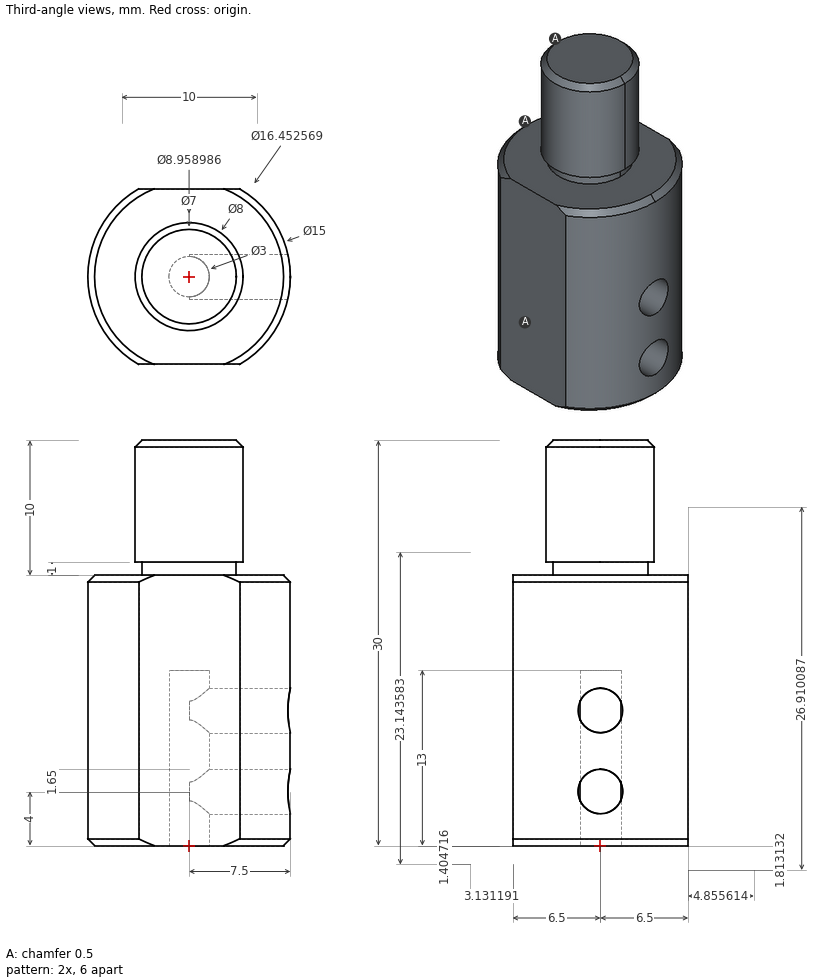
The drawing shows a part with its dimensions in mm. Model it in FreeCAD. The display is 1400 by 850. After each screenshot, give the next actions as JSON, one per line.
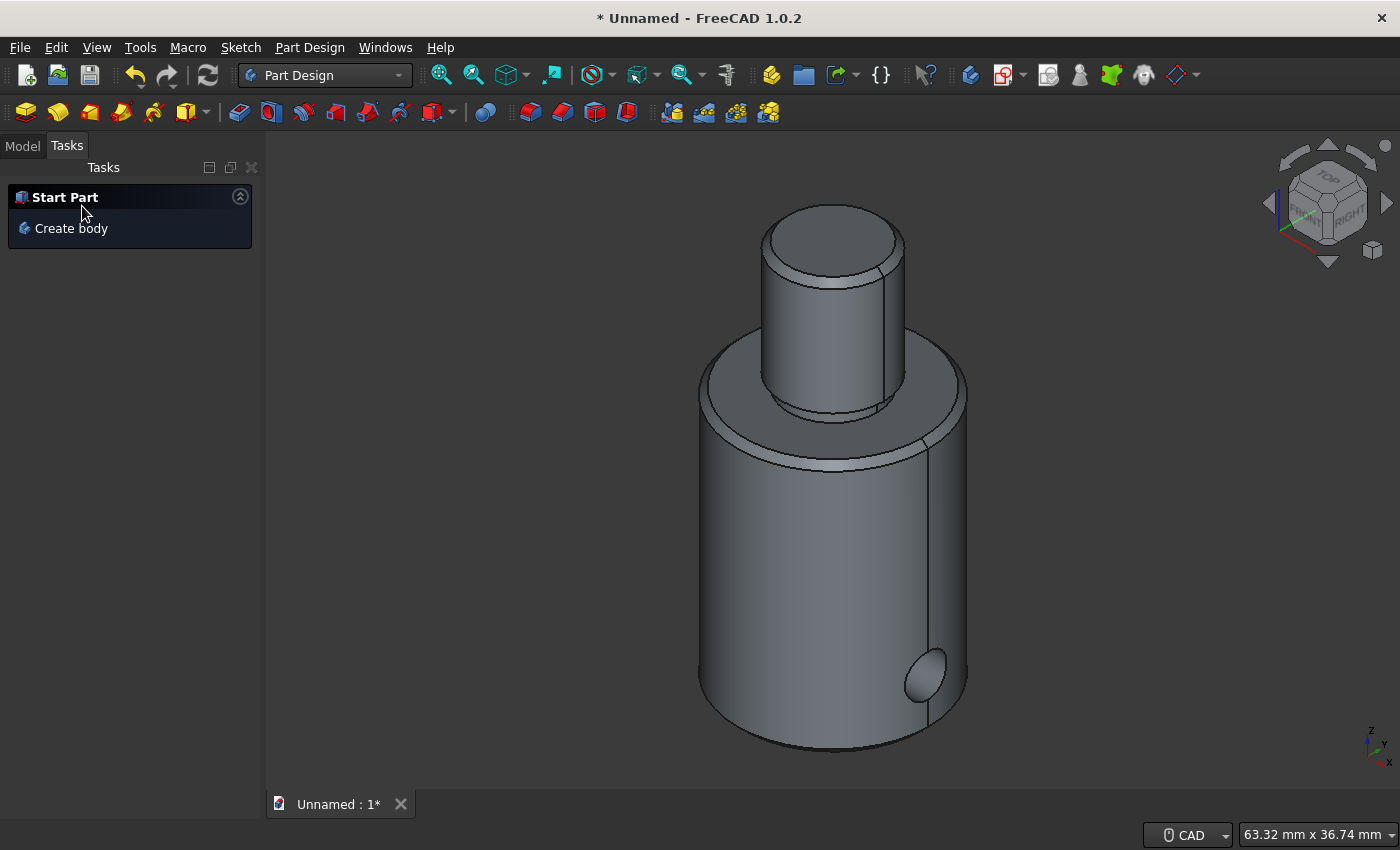
{"action": "left_click", "coordinate": [442, 76]}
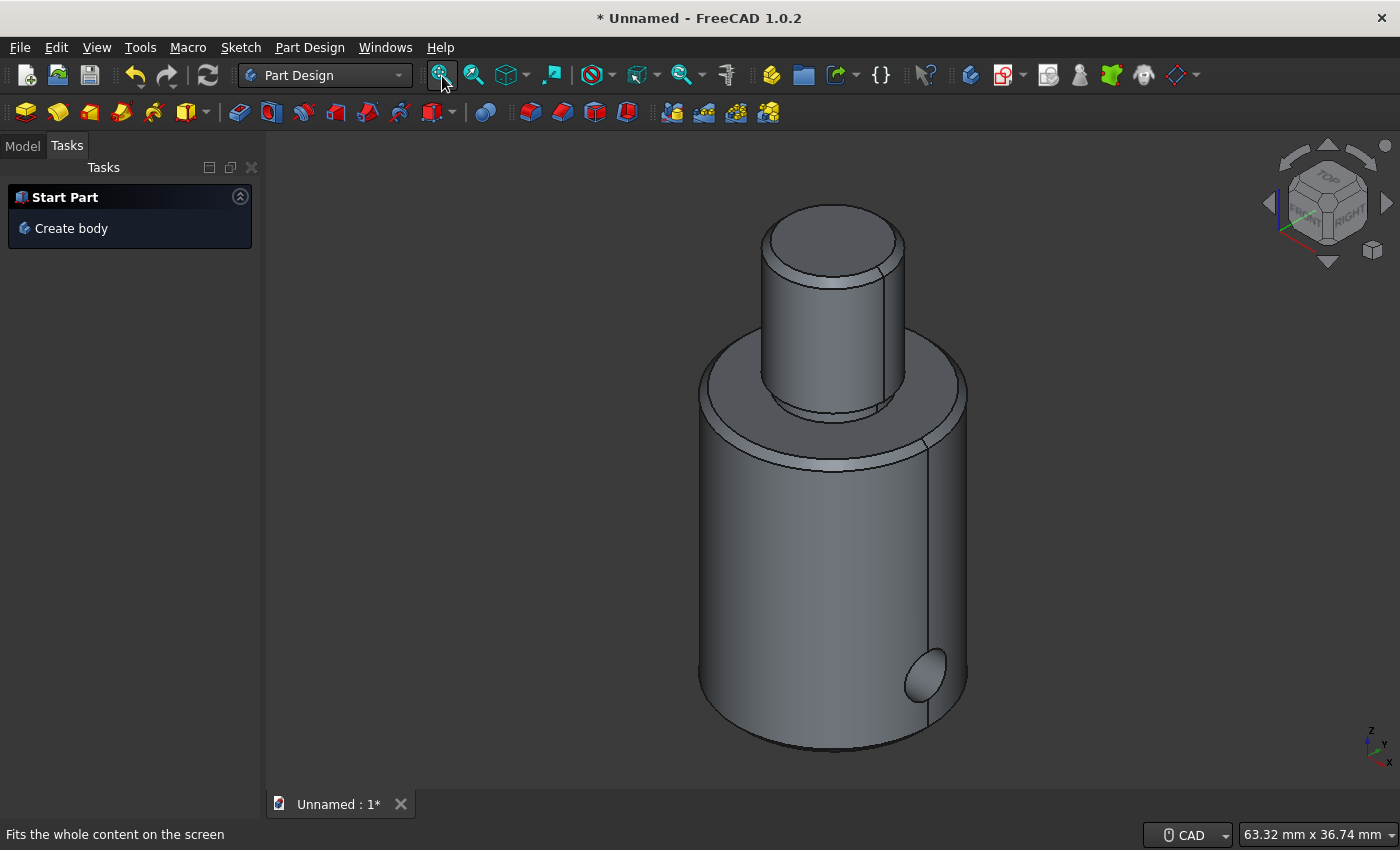
{"action": "left_click", "coordinate": [23, 145]}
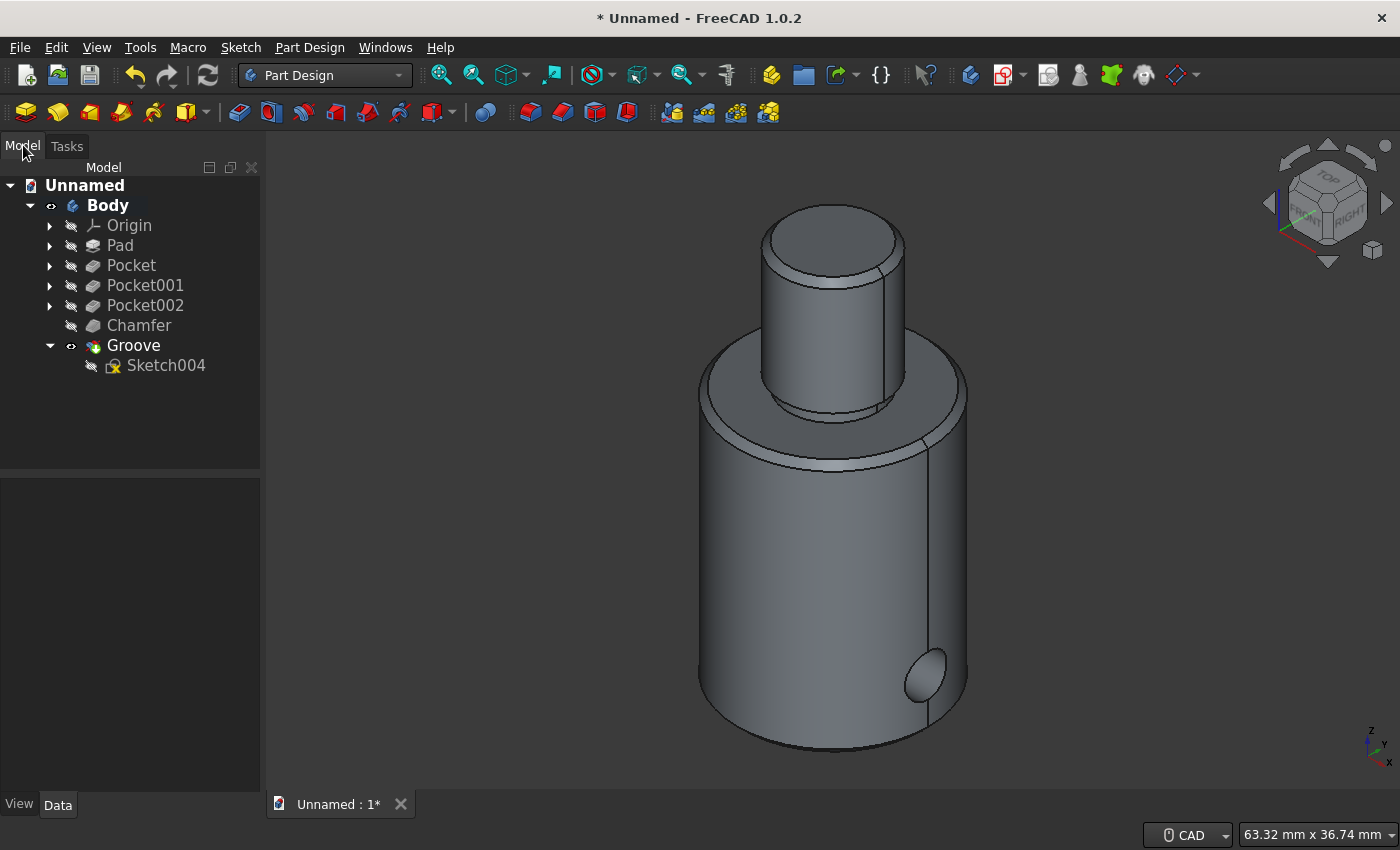
{"action": "left_click", "coordinate": [116, 346]}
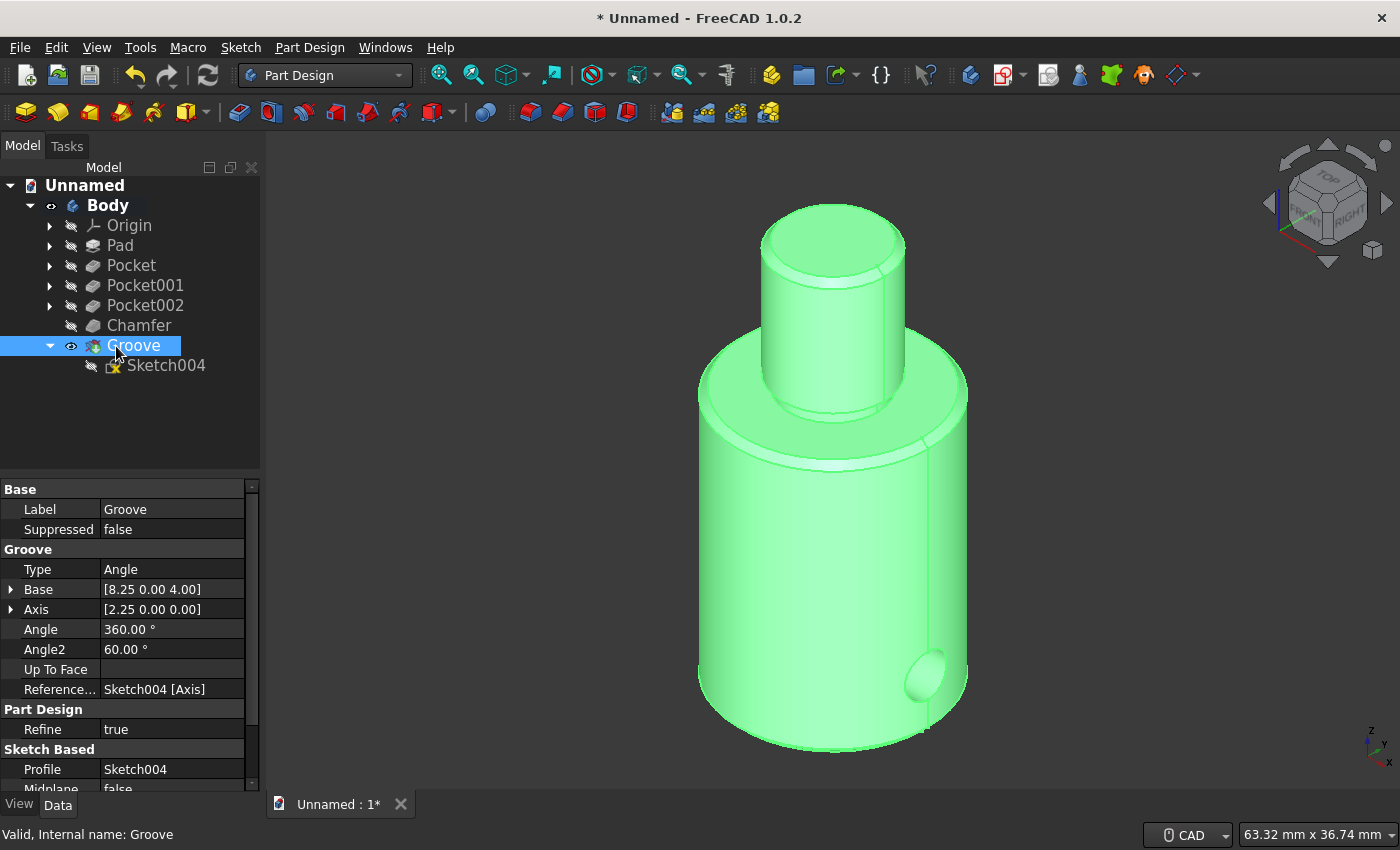
{"action": "left_click", "coordinate": [704, 112]}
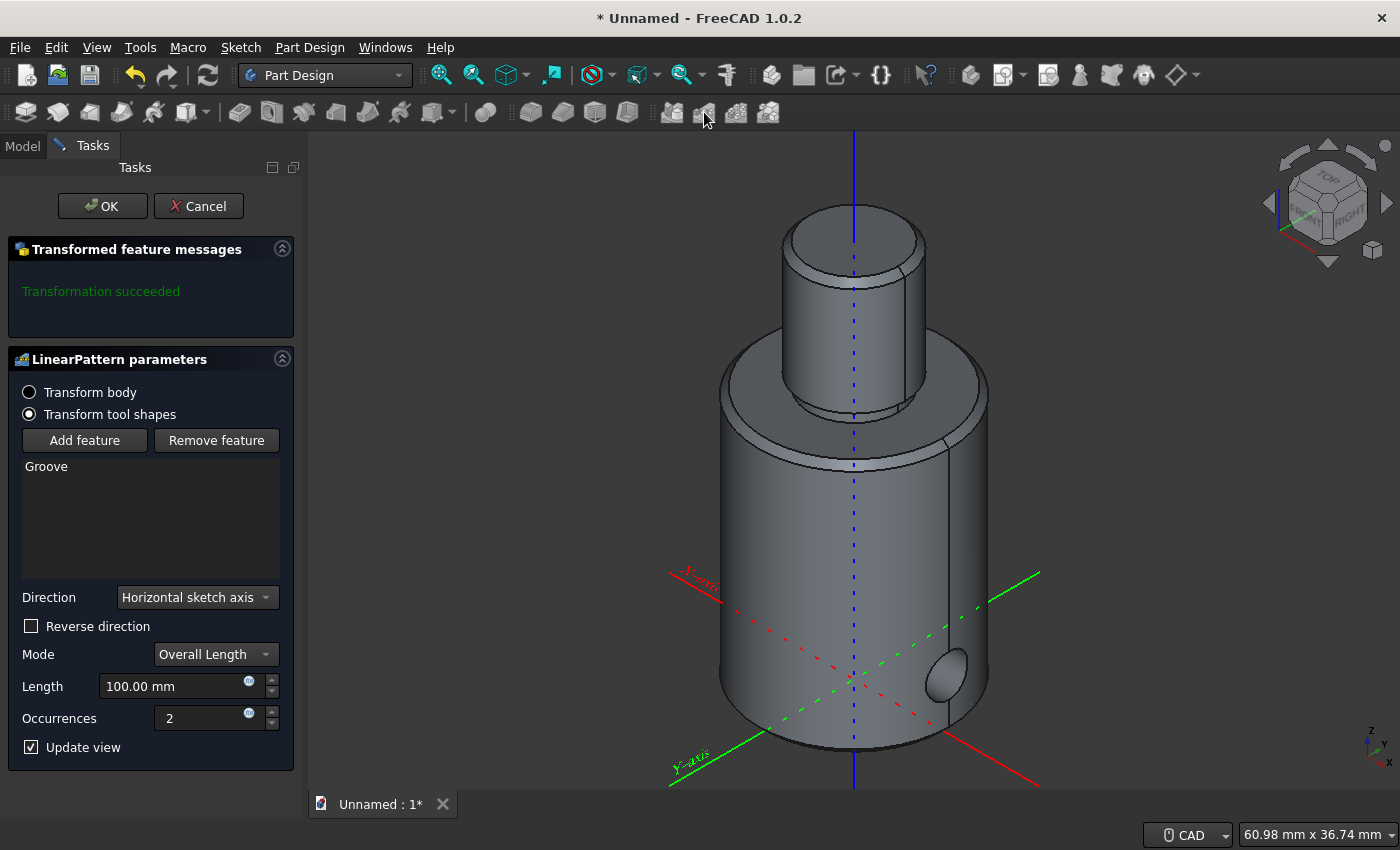
{"action": "left_click", "coordinate": [198, 598]}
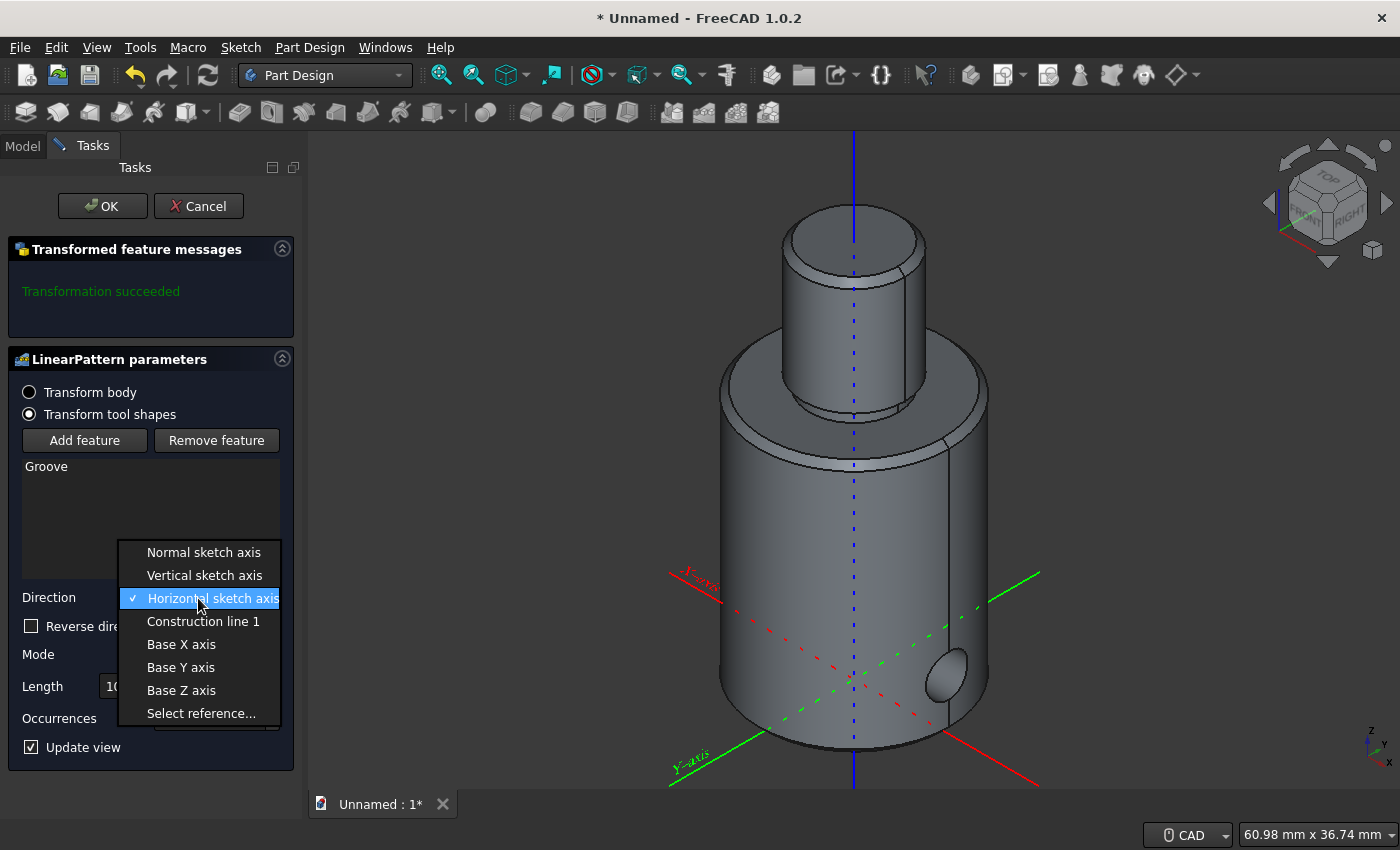
{"action": "left_click", "coordinate": [198, 690]}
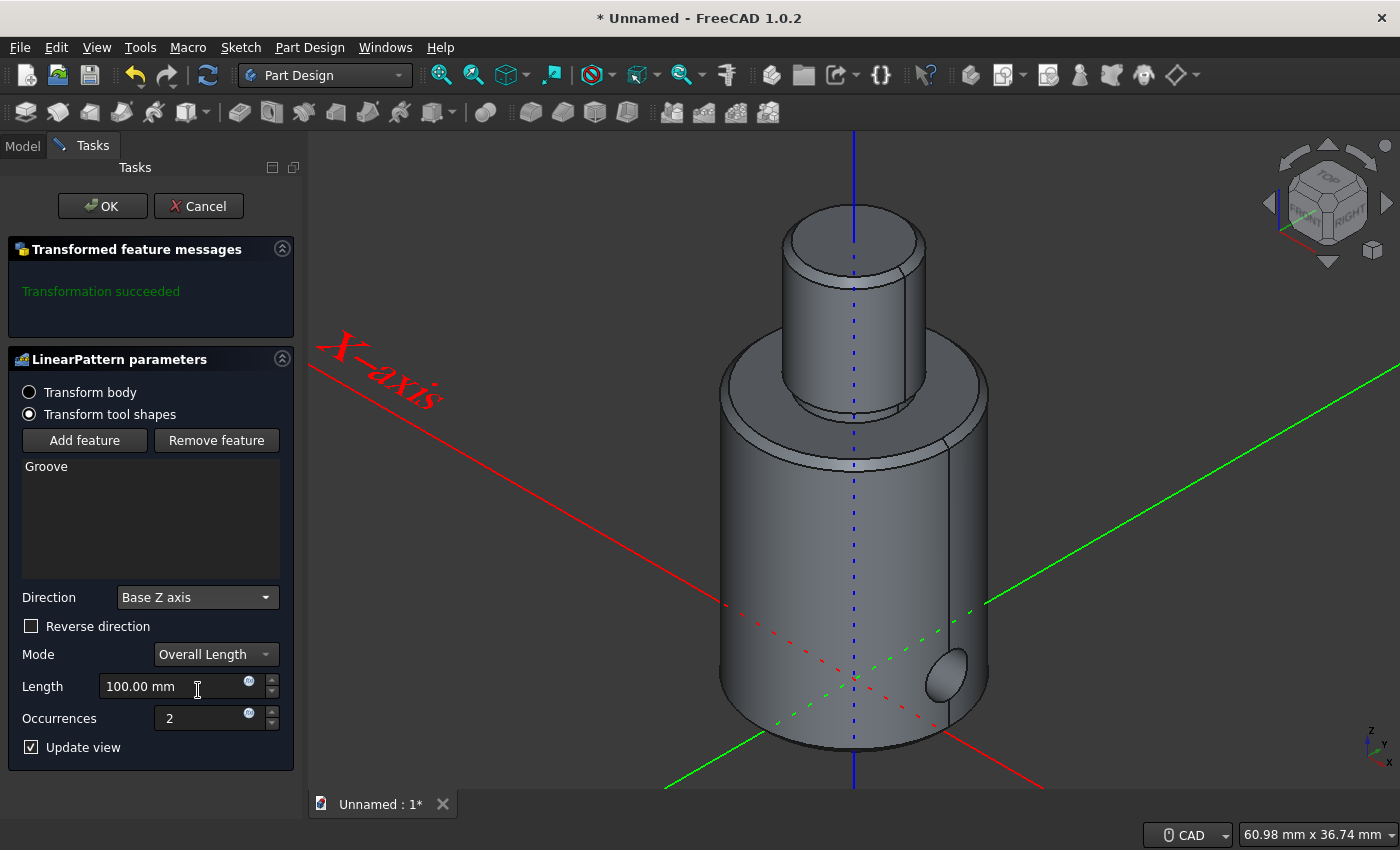
{"action": "left_click", "coordinate": [217, 654]}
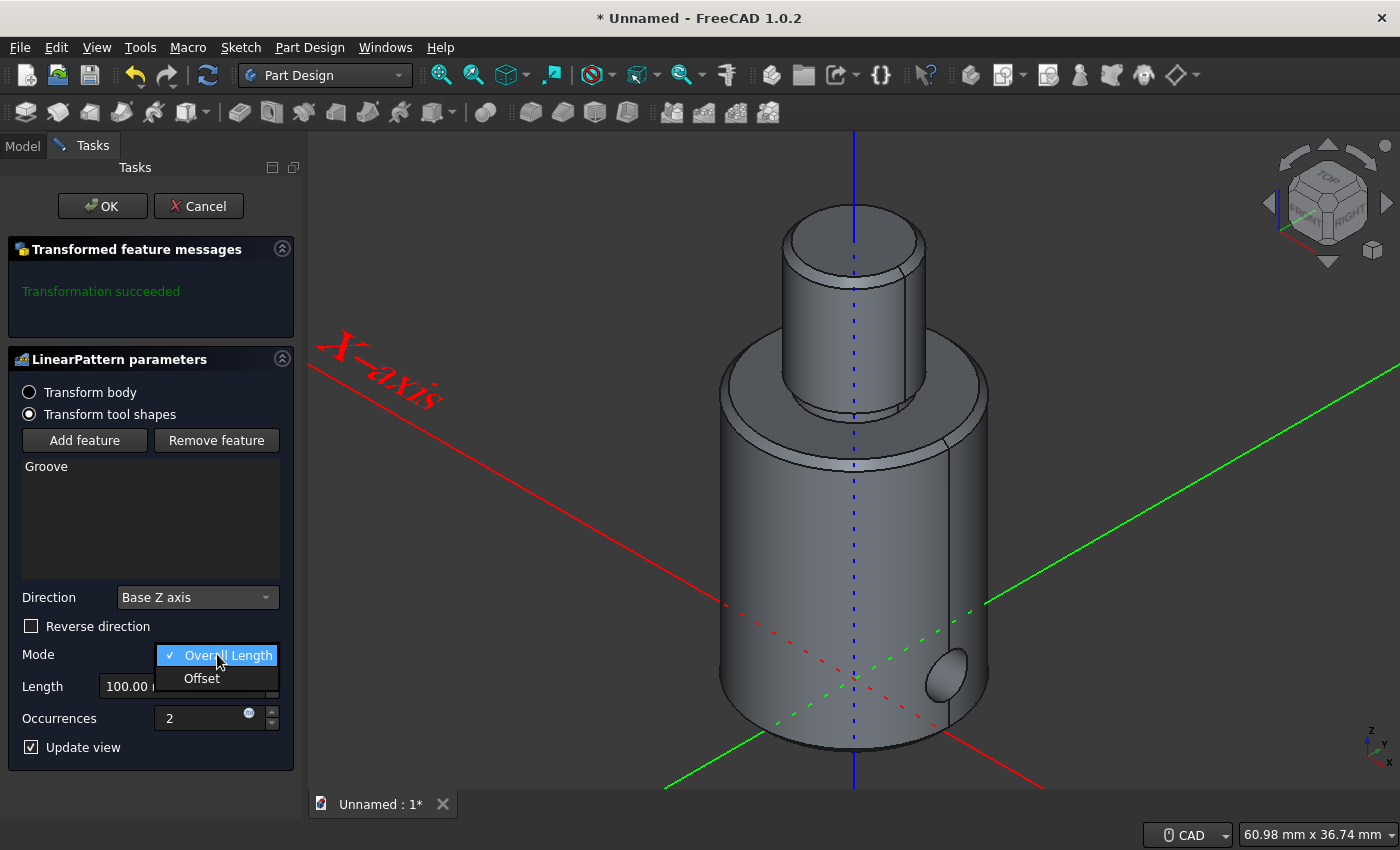
{"action": "left_click", "coordinate": [216, 678]}